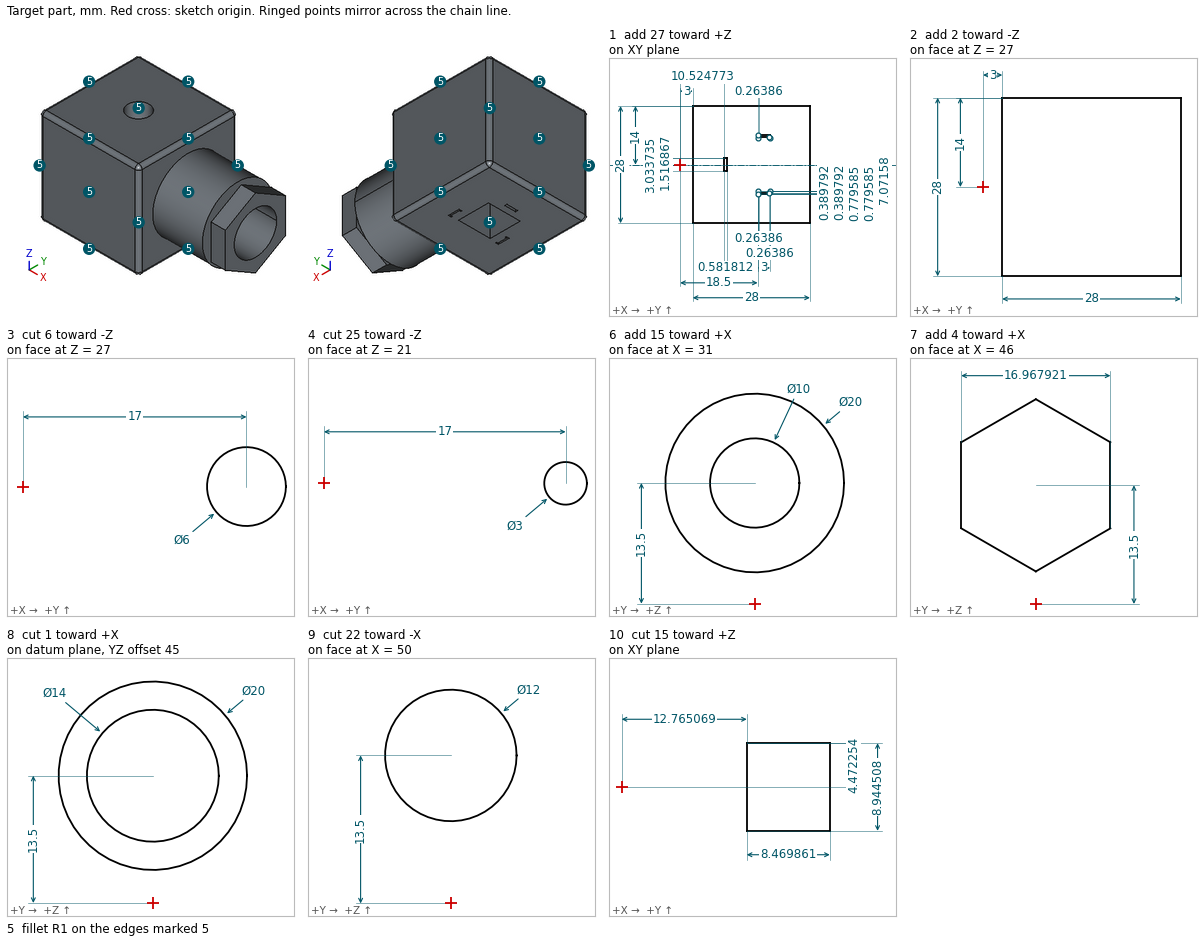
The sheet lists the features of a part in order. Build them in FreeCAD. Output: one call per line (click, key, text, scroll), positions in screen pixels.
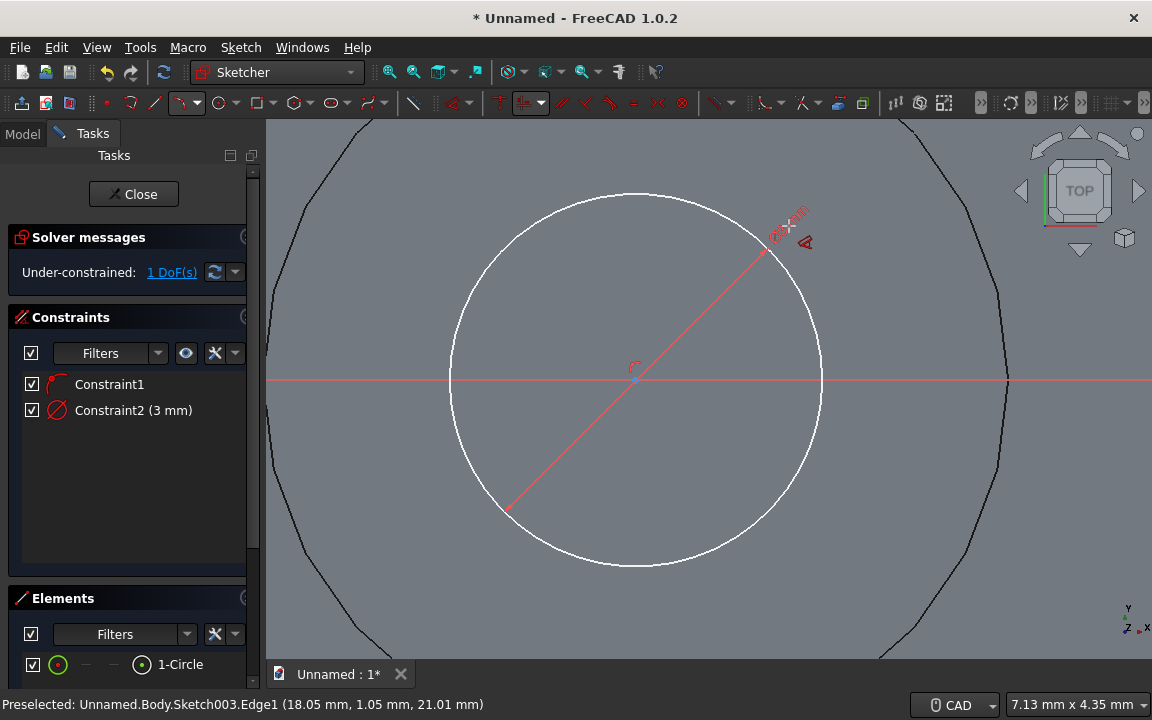
click(636, 380)
click(386, 414)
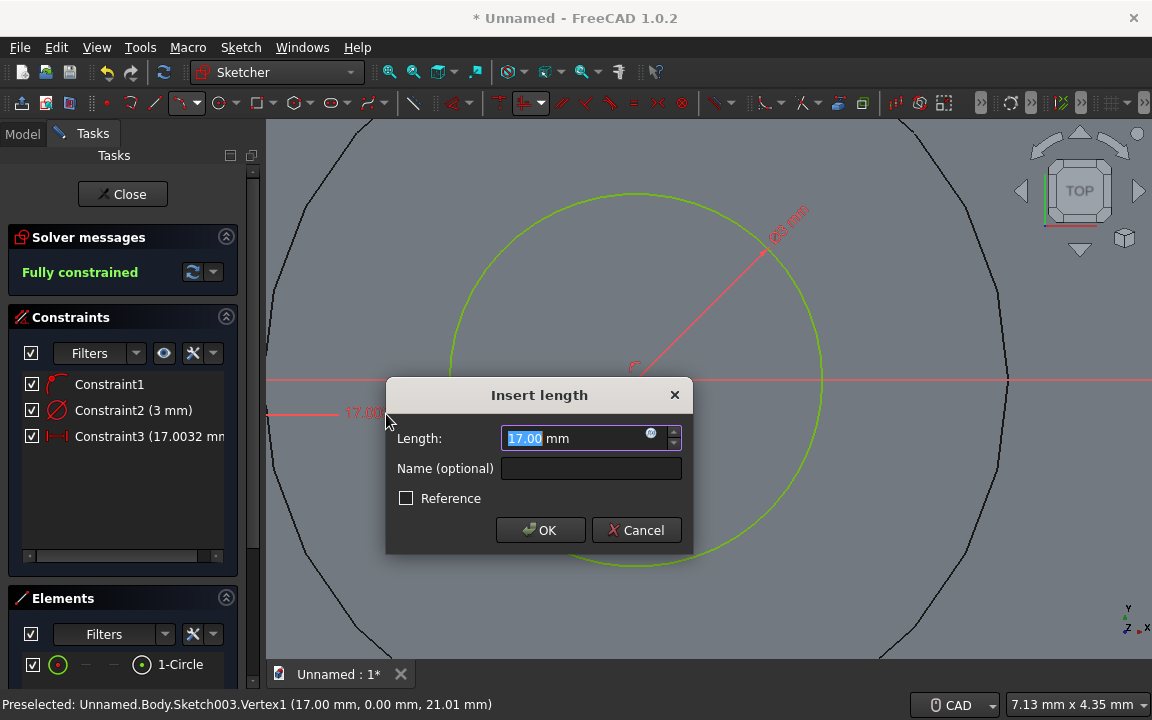
text(17)
key(Return)
key(Escape)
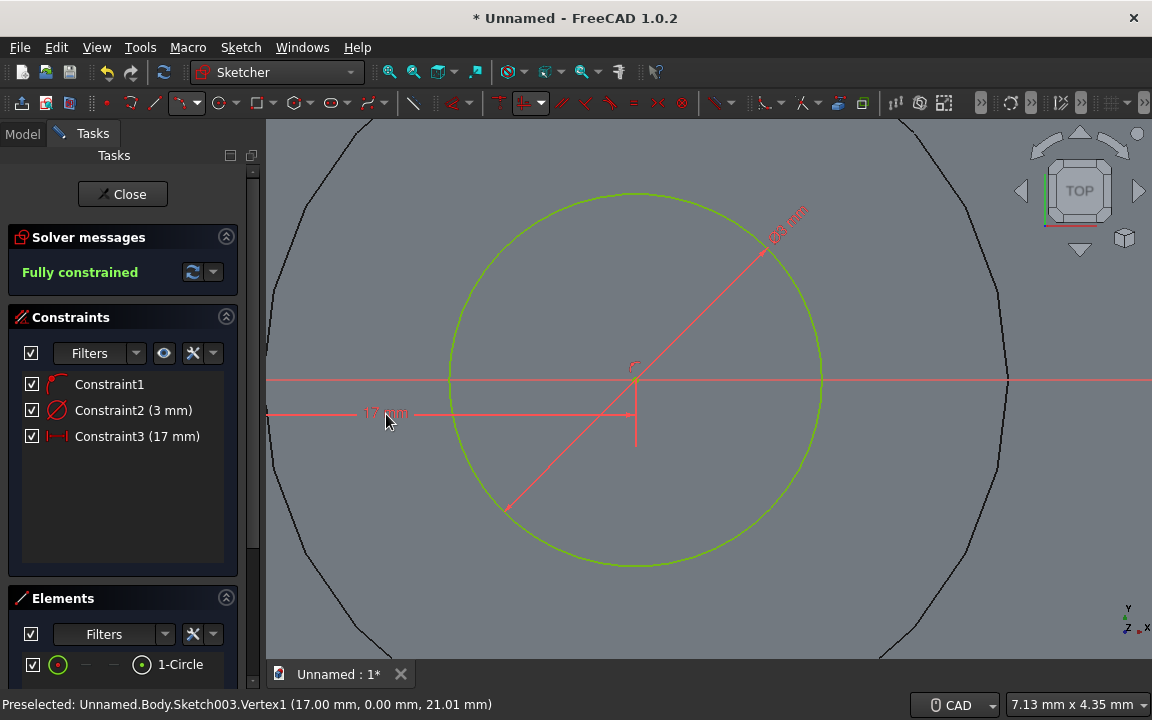
click(123, 194)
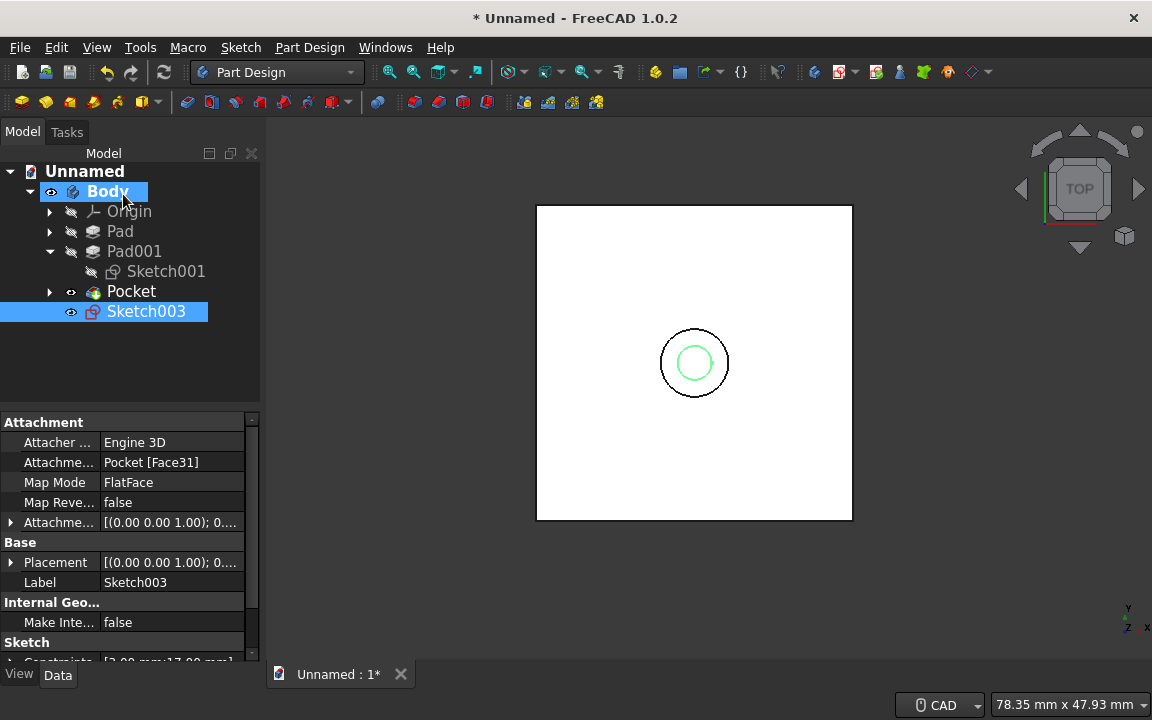
click(188, 102)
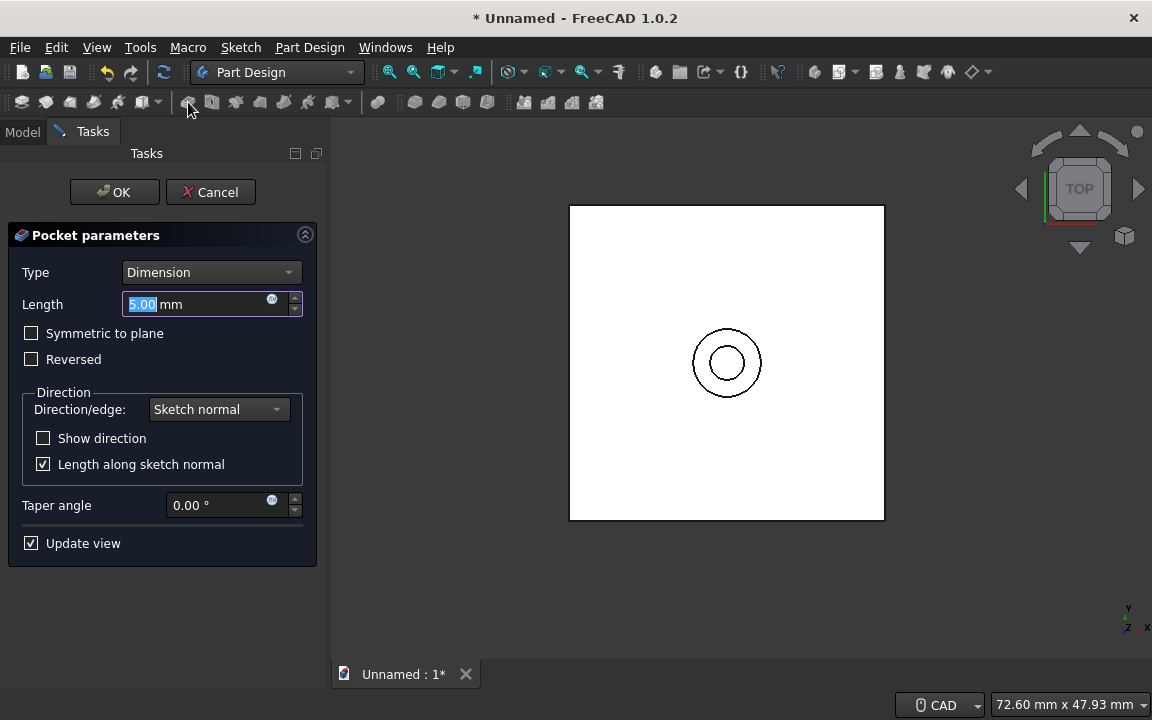
text(25)
key(Tab)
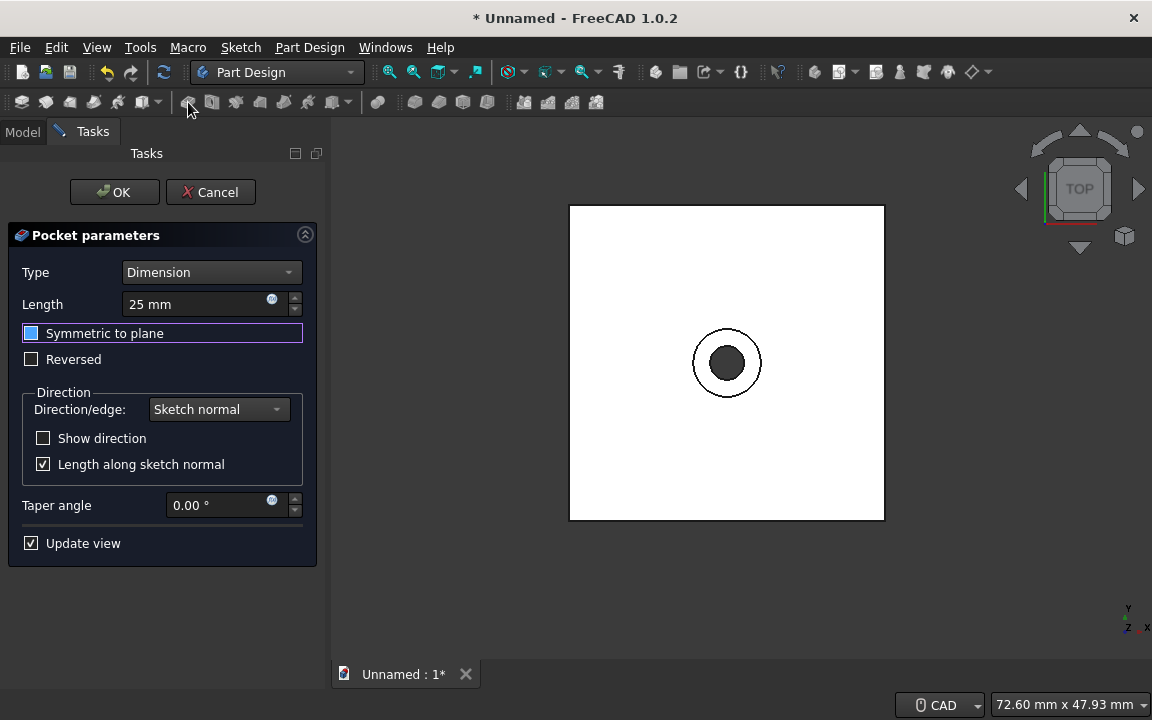
click(115, 192)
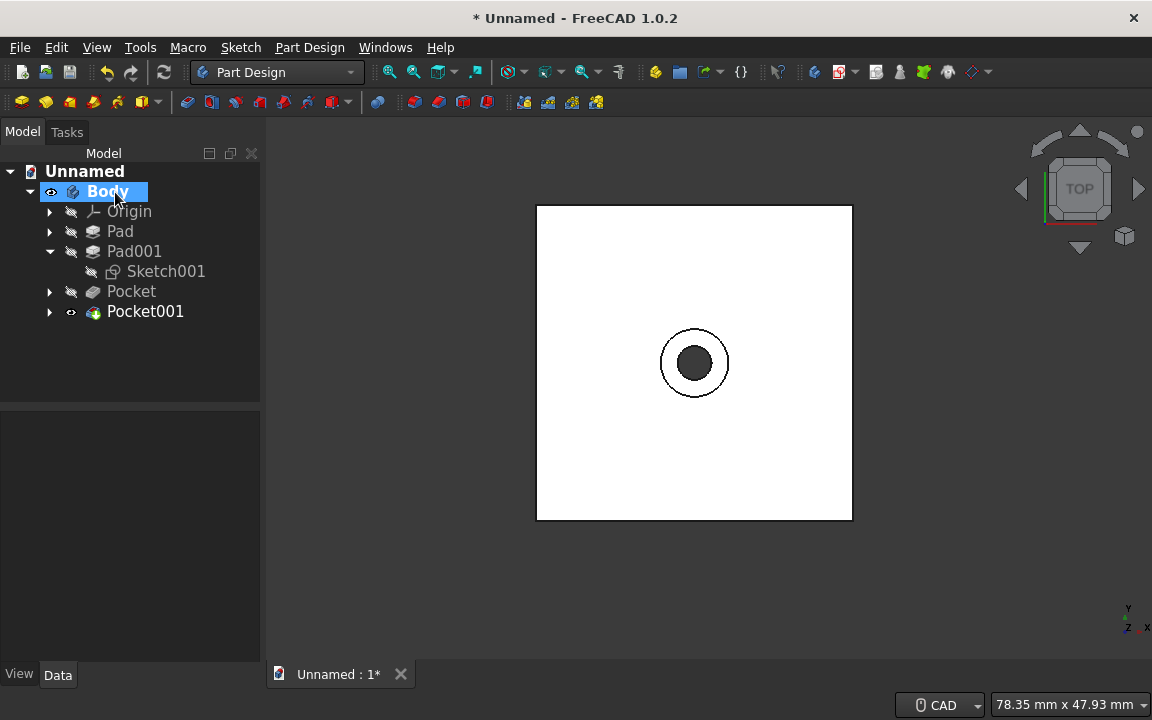
click(853, 362)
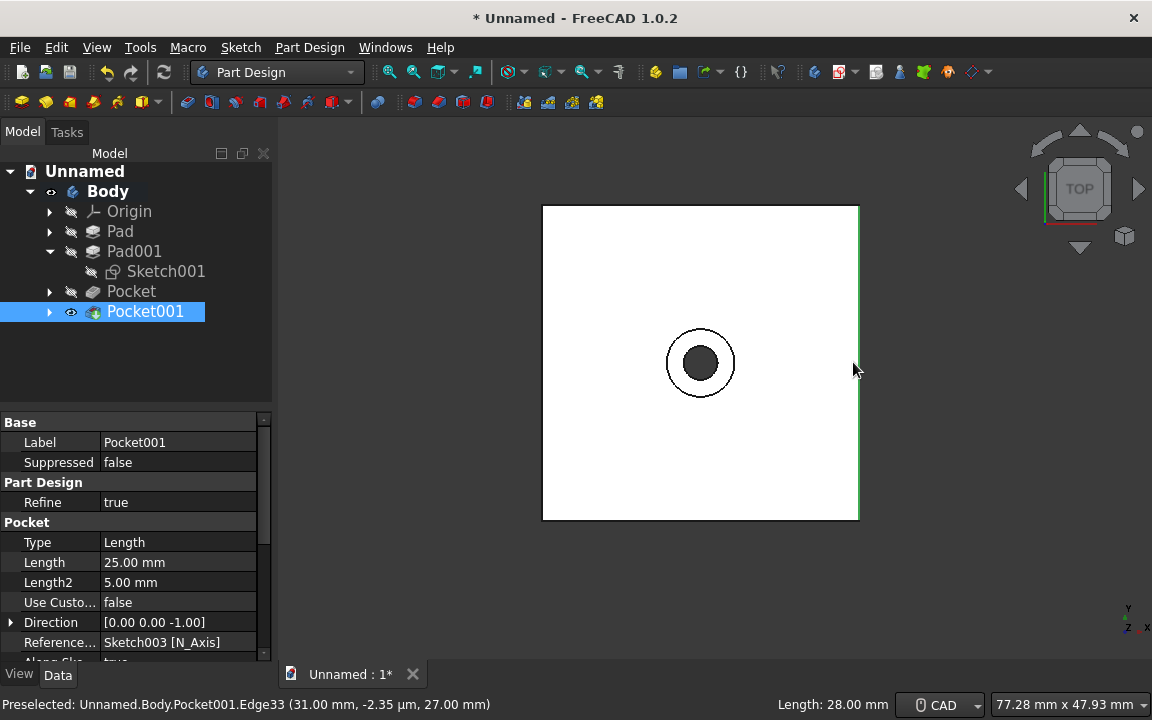
key(0)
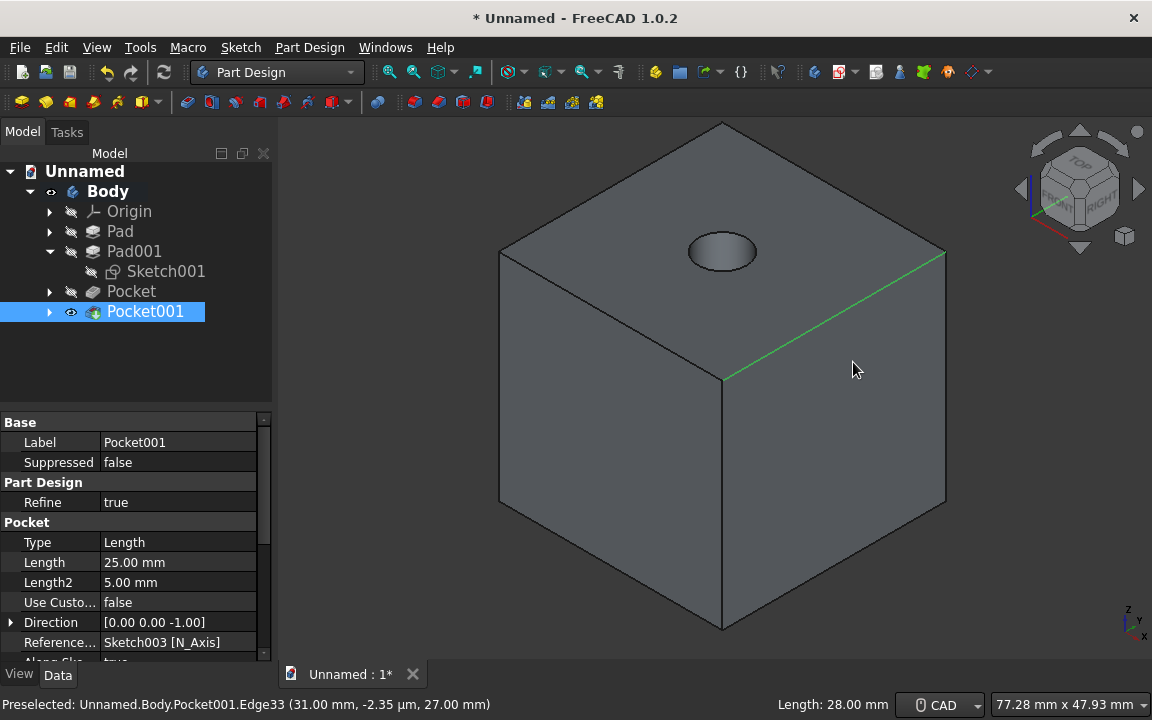
click(611, 440, ctrl)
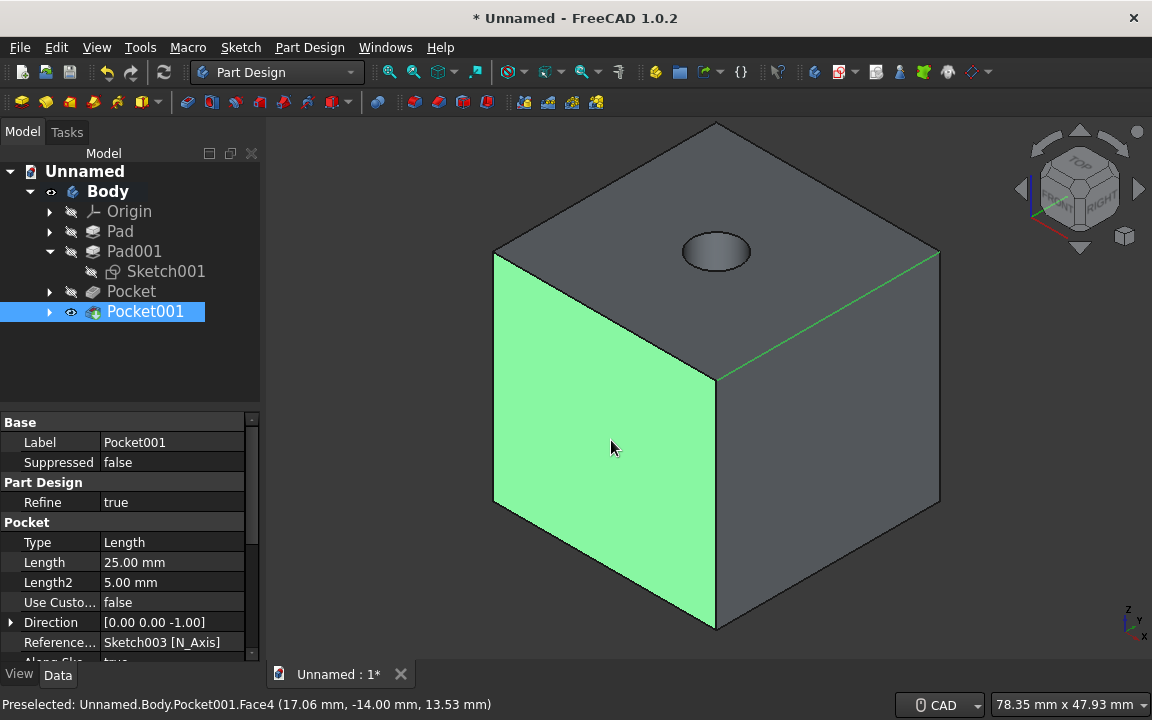
key(2)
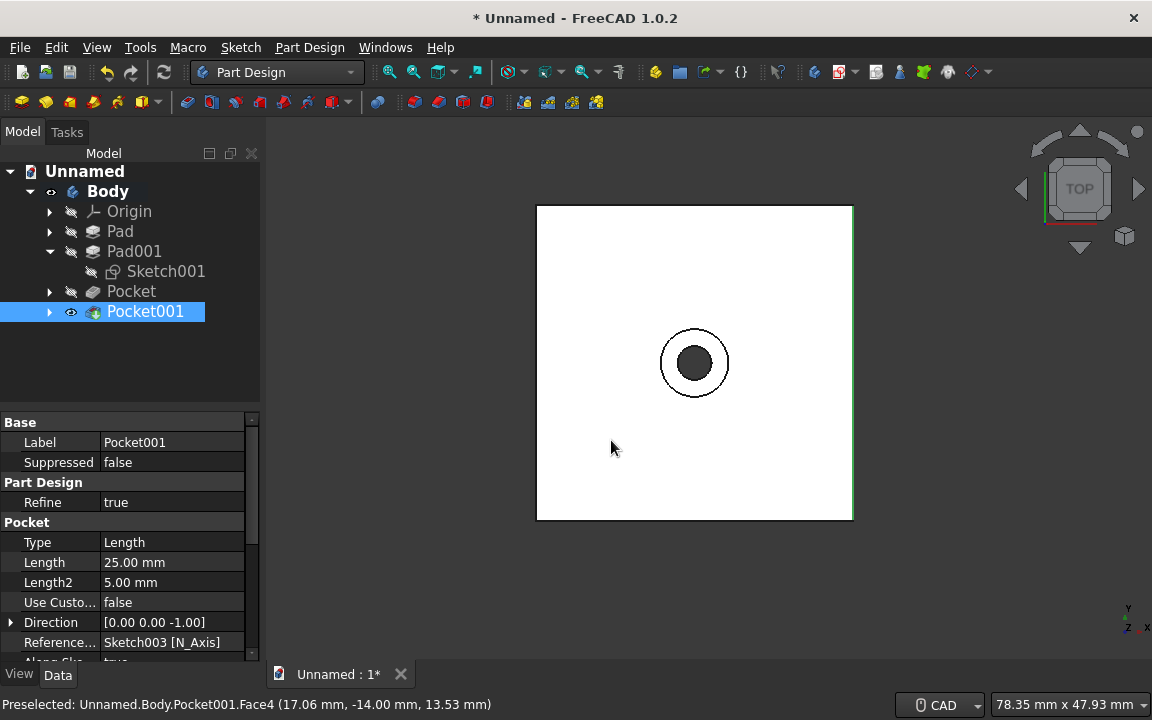
key(1)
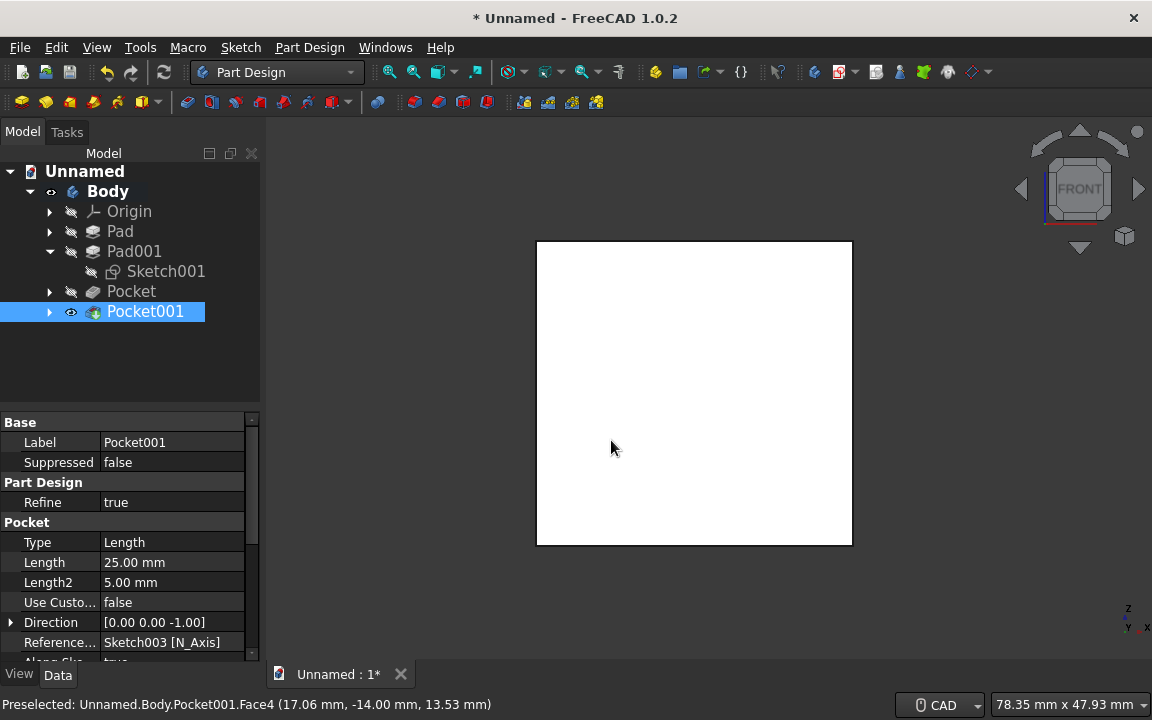
key(3)